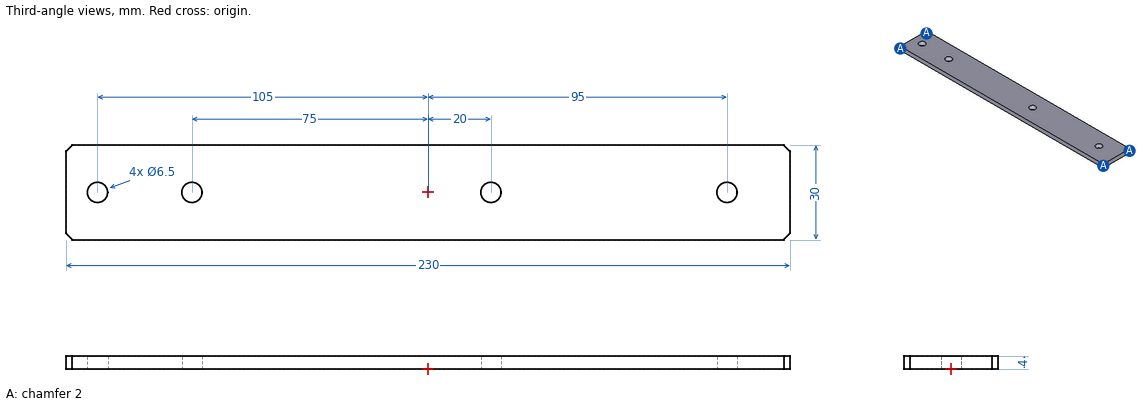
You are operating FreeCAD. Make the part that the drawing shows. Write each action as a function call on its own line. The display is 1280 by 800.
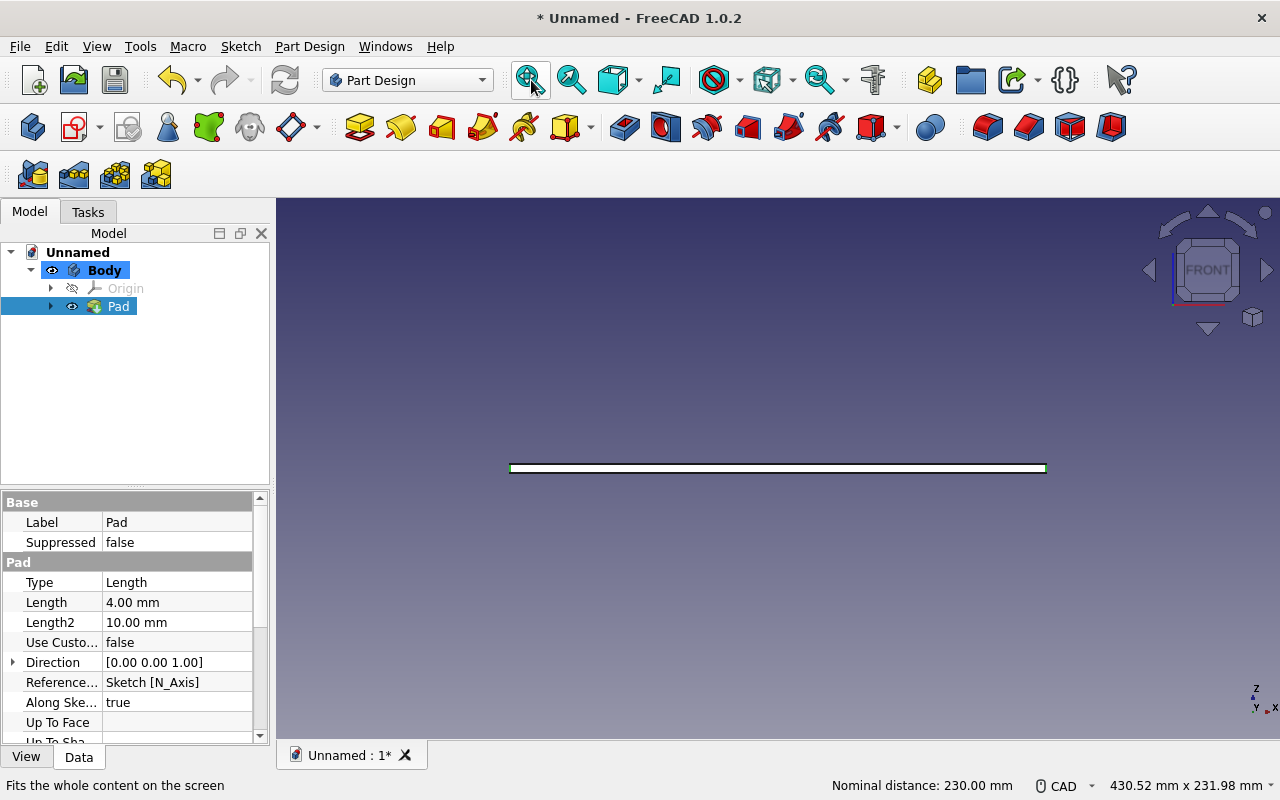
key(3)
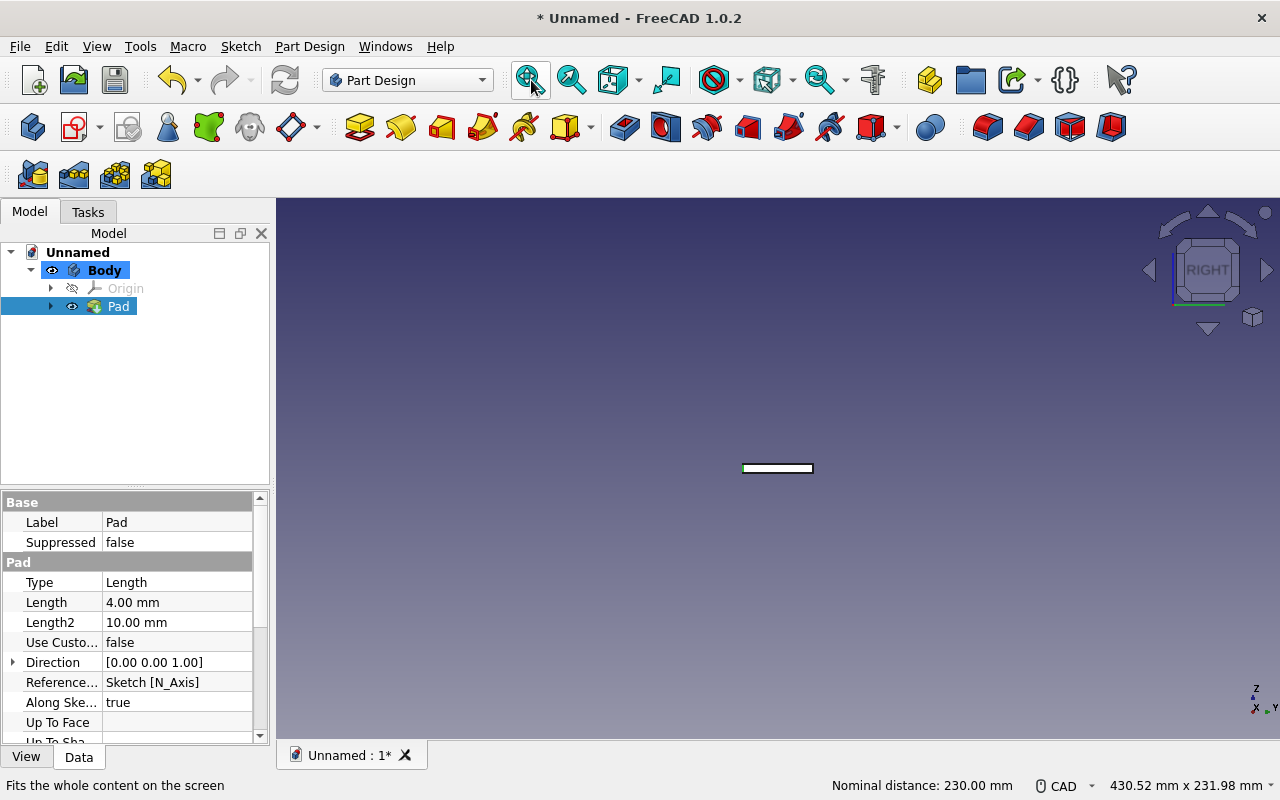
click(531, 80)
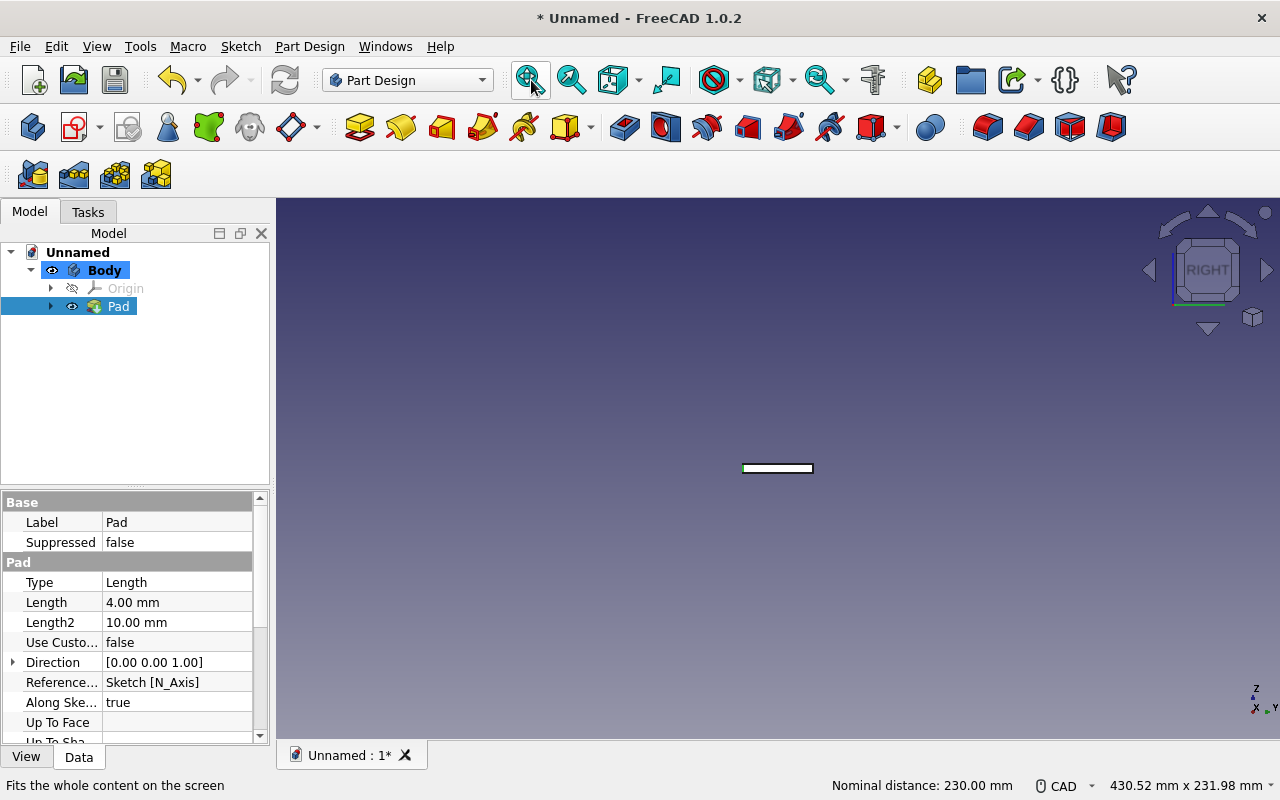
scroll(813, 467, up, 8)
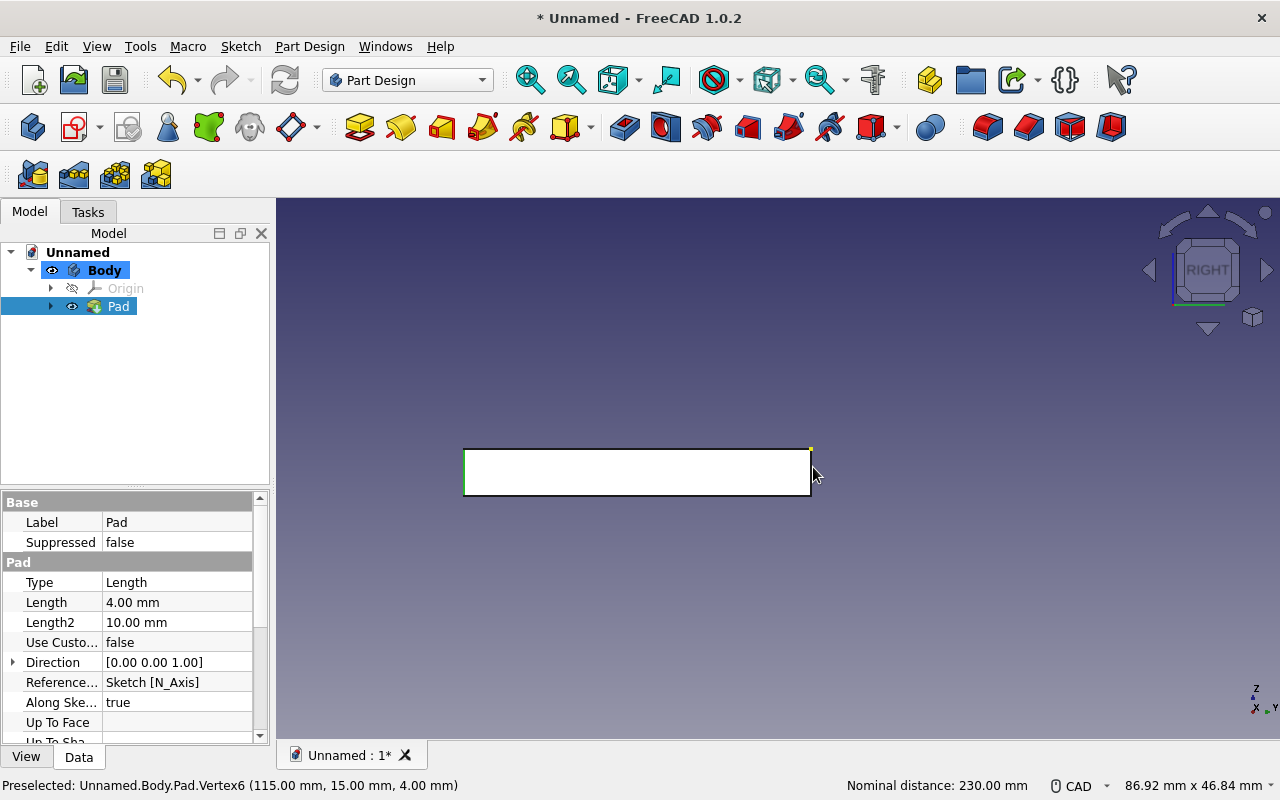
click(811, 471, ctrl)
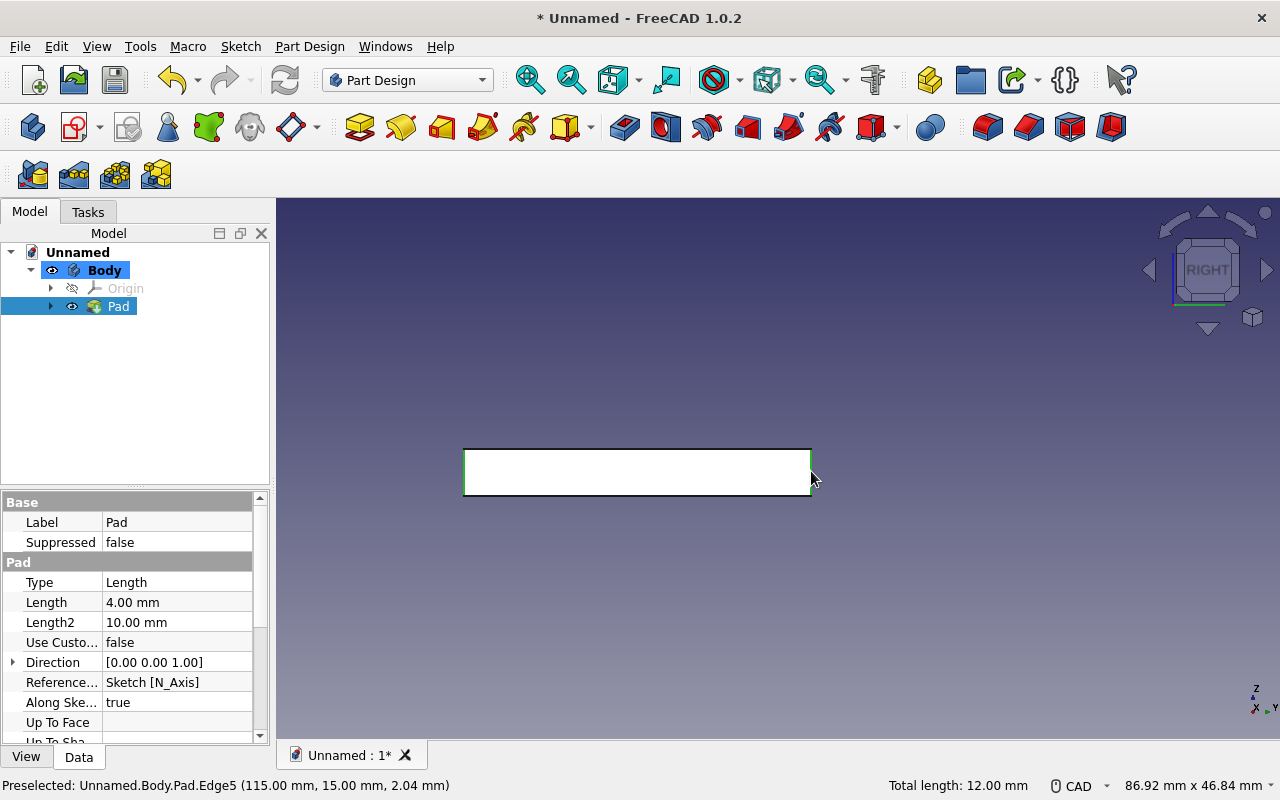
click(531, 80)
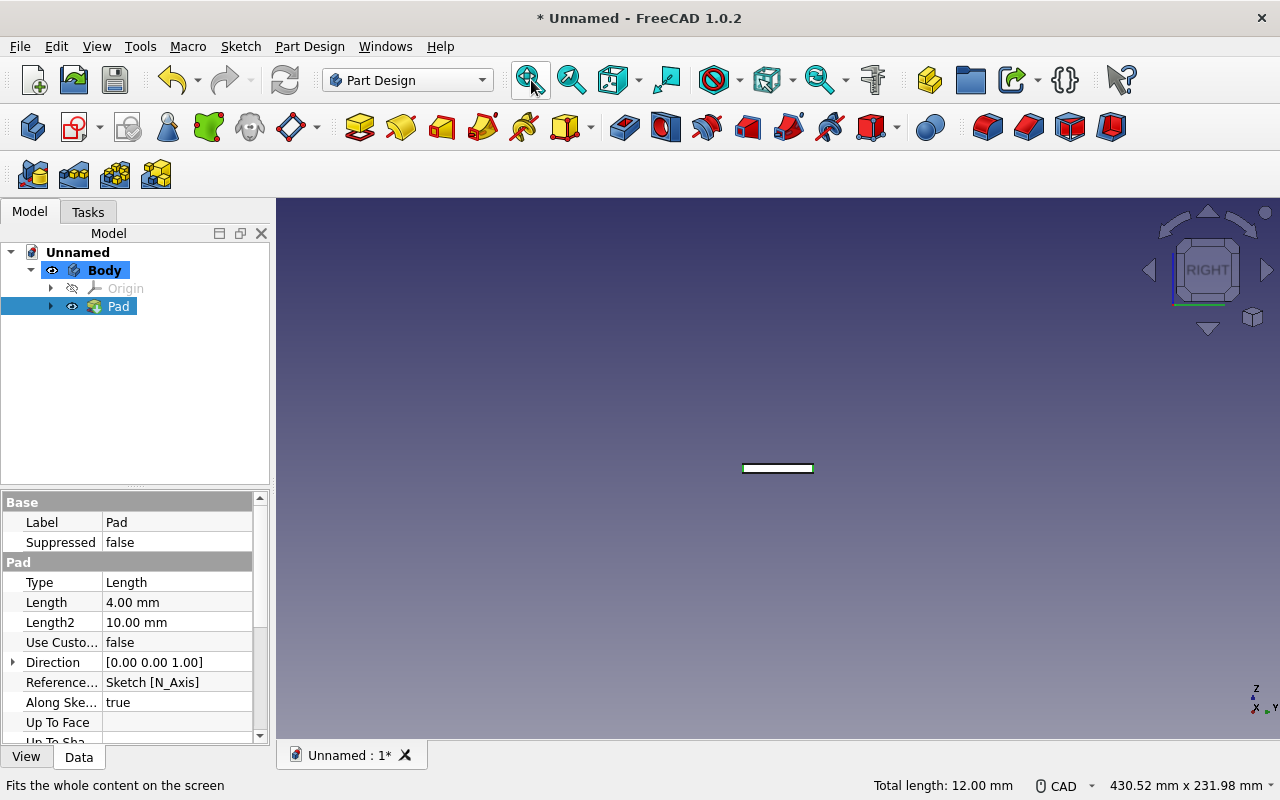
key(5)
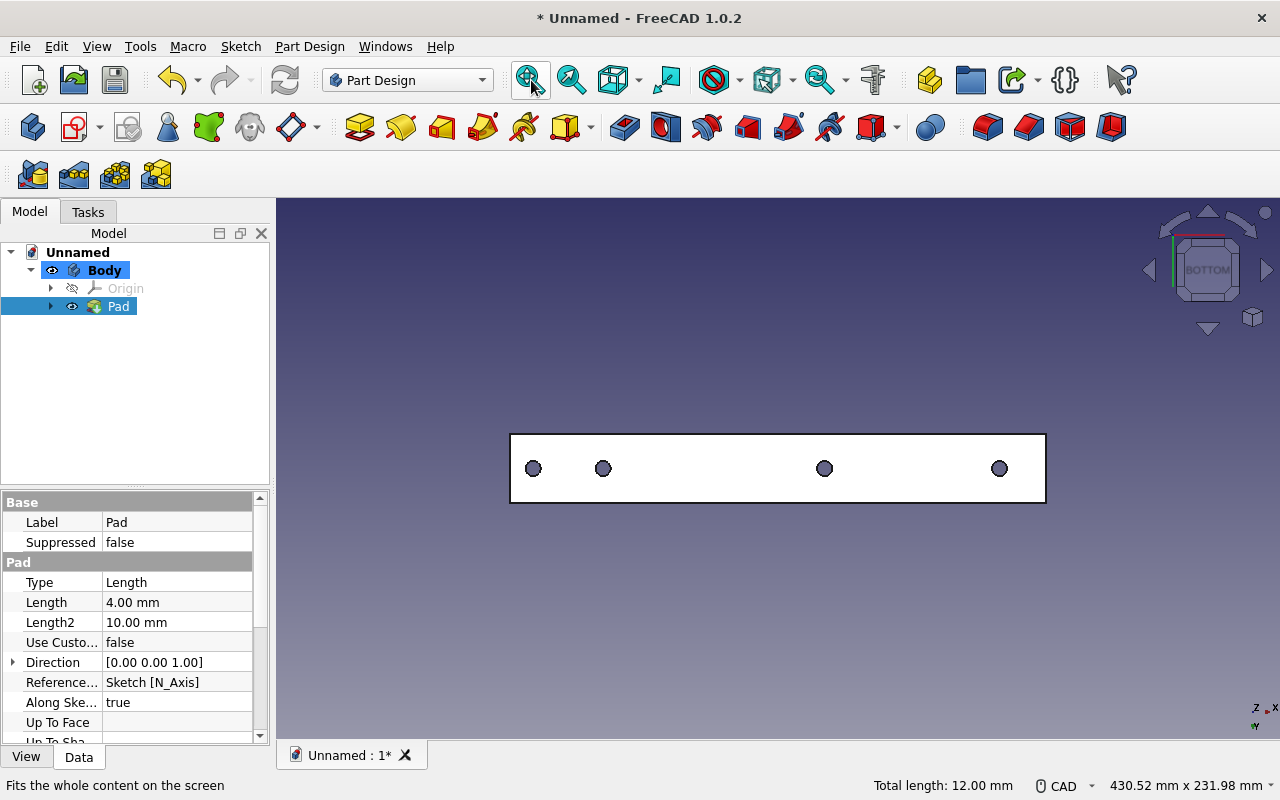
scroll(510, 502, up, 8)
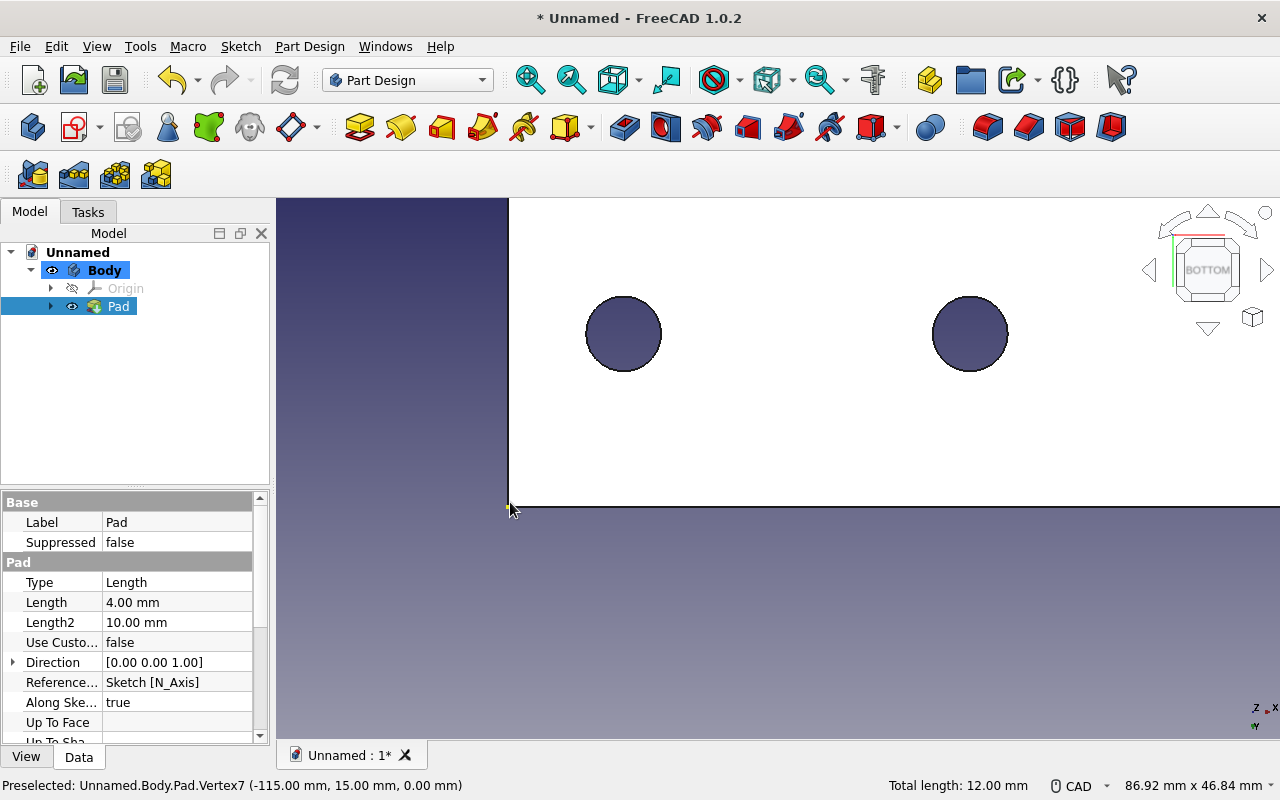
key(v)
key(f)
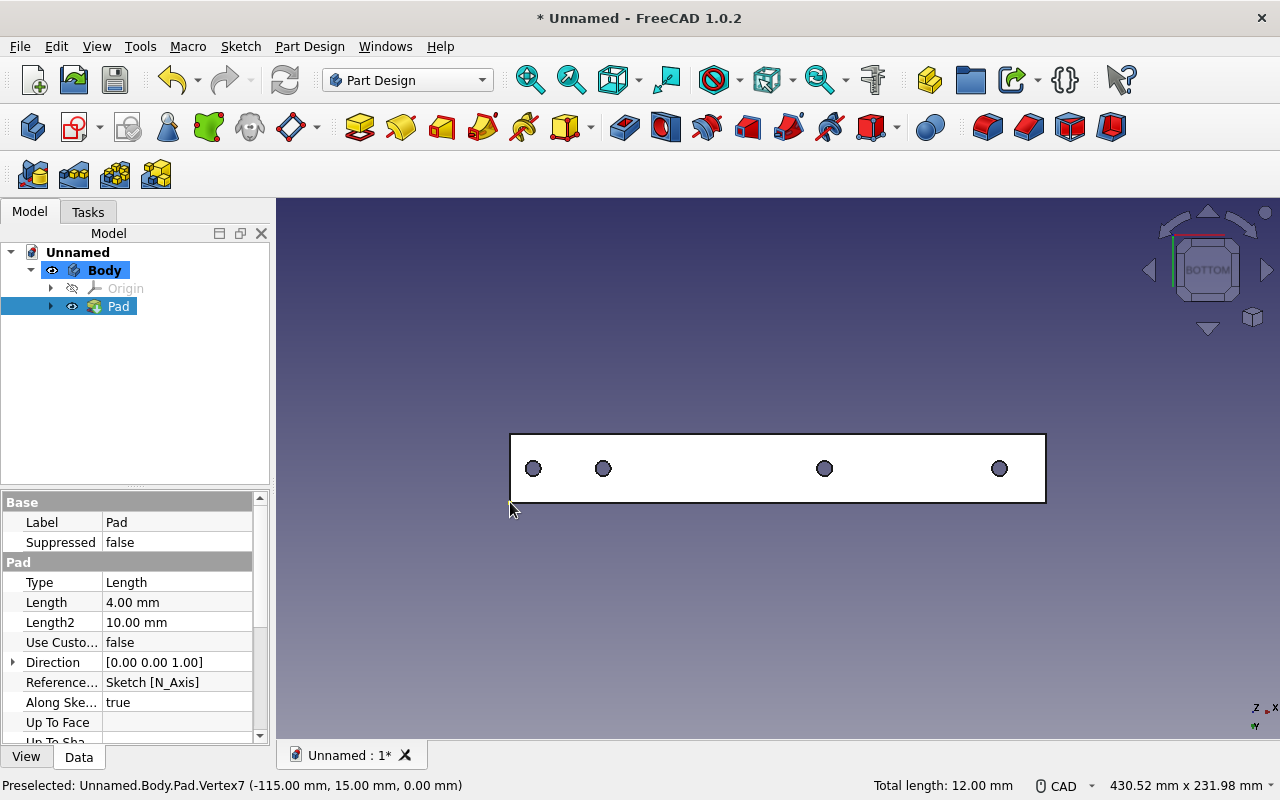
key(4)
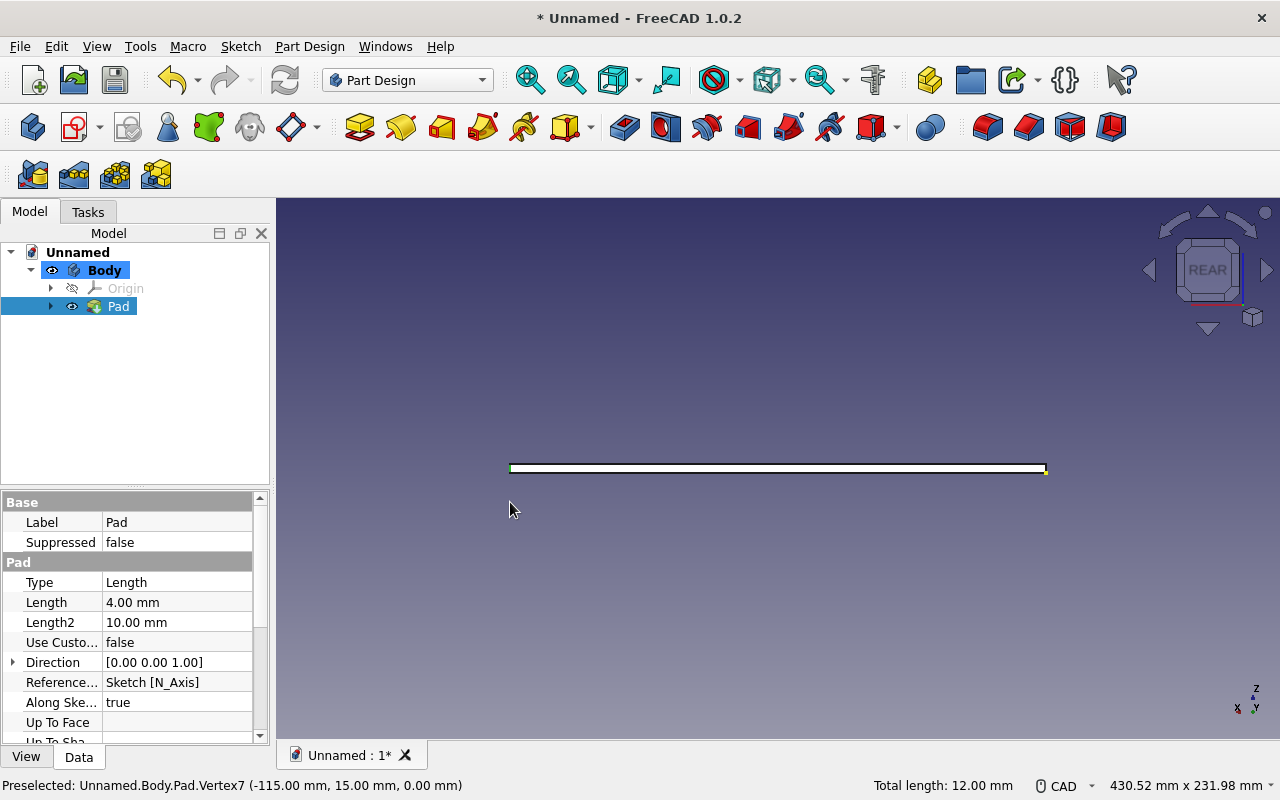
scroll(1046, 468, up, 8)